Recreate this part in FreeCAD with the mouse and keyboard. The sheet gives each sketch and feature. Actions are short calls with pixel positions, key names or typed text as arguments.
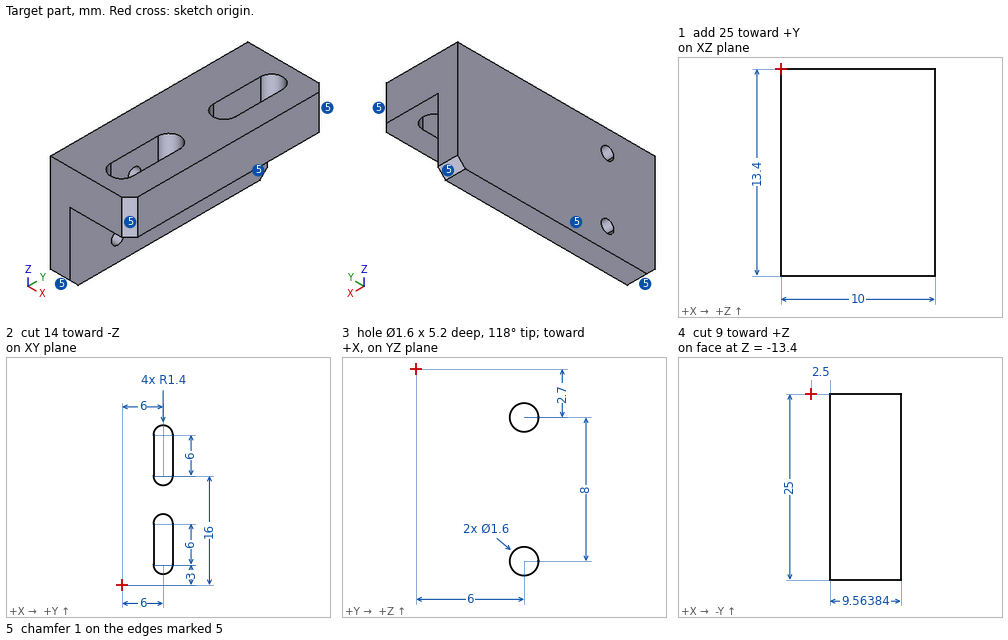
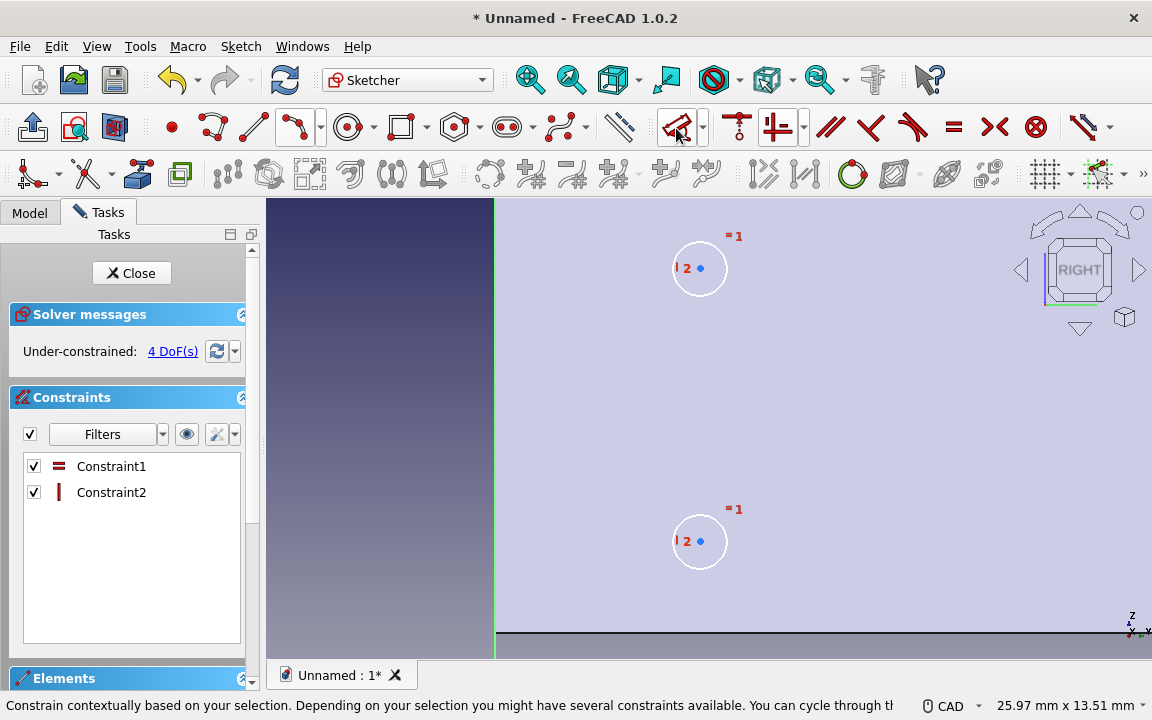
click(719, 523)
click(742, 500)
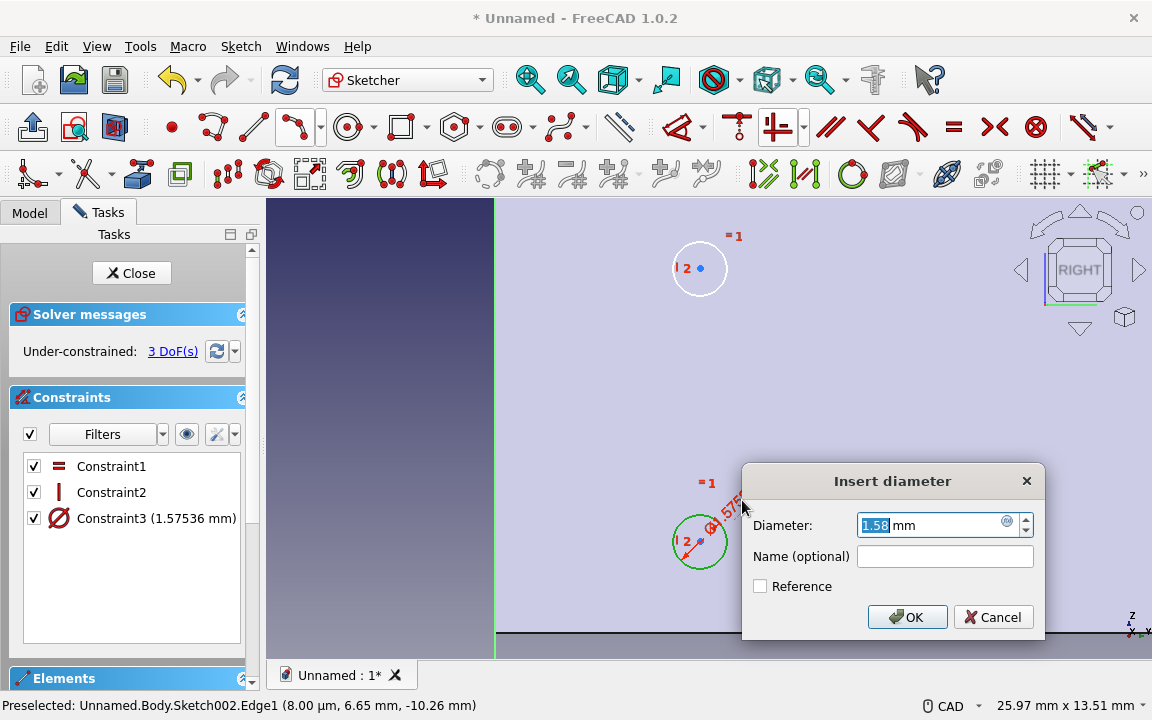
text(1.6)
key(Return)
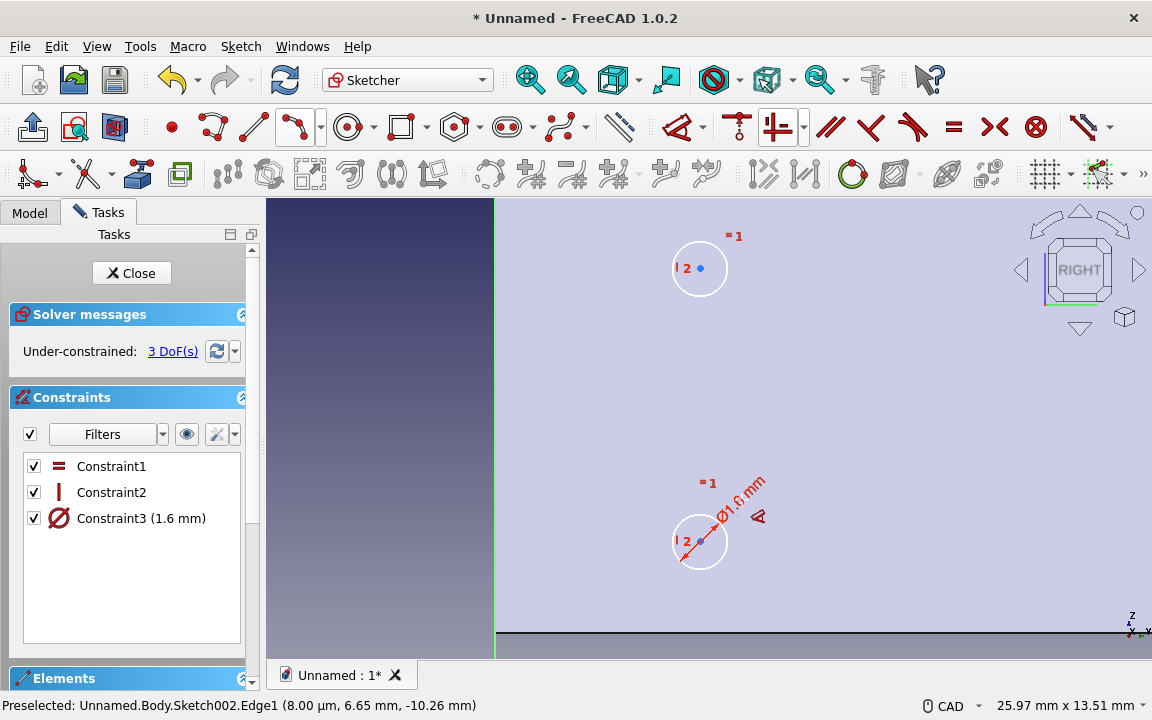
click(700, 542)
click(598, 576)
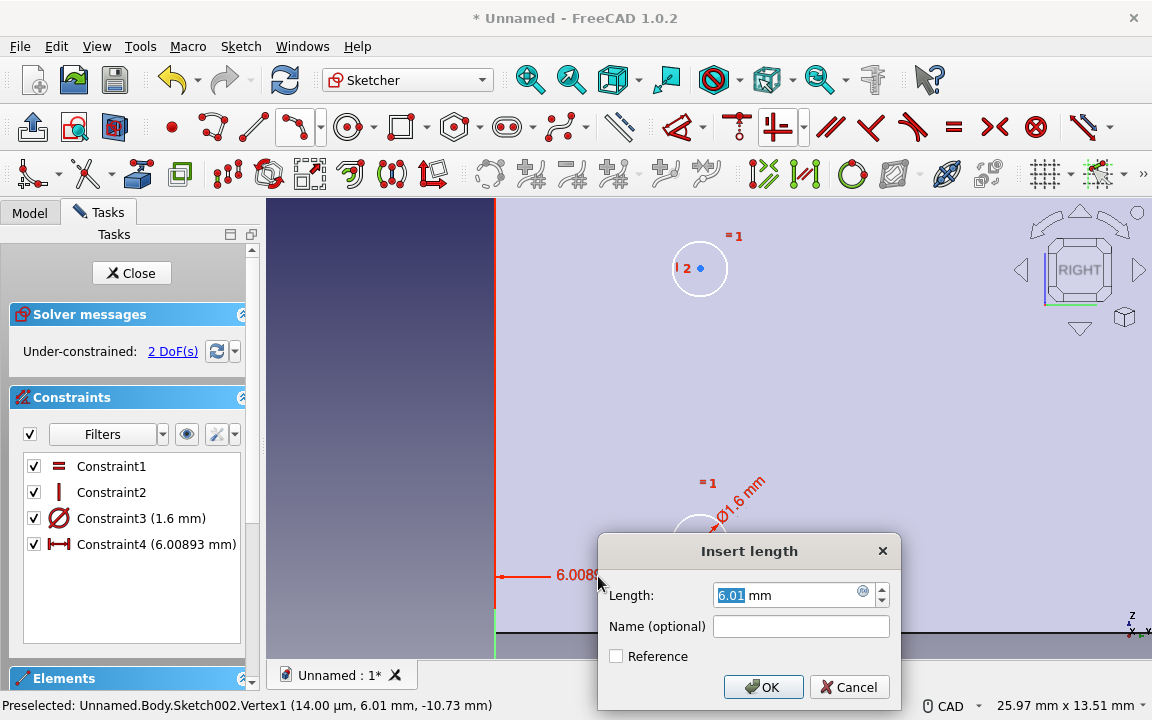
text(6)
key(Return)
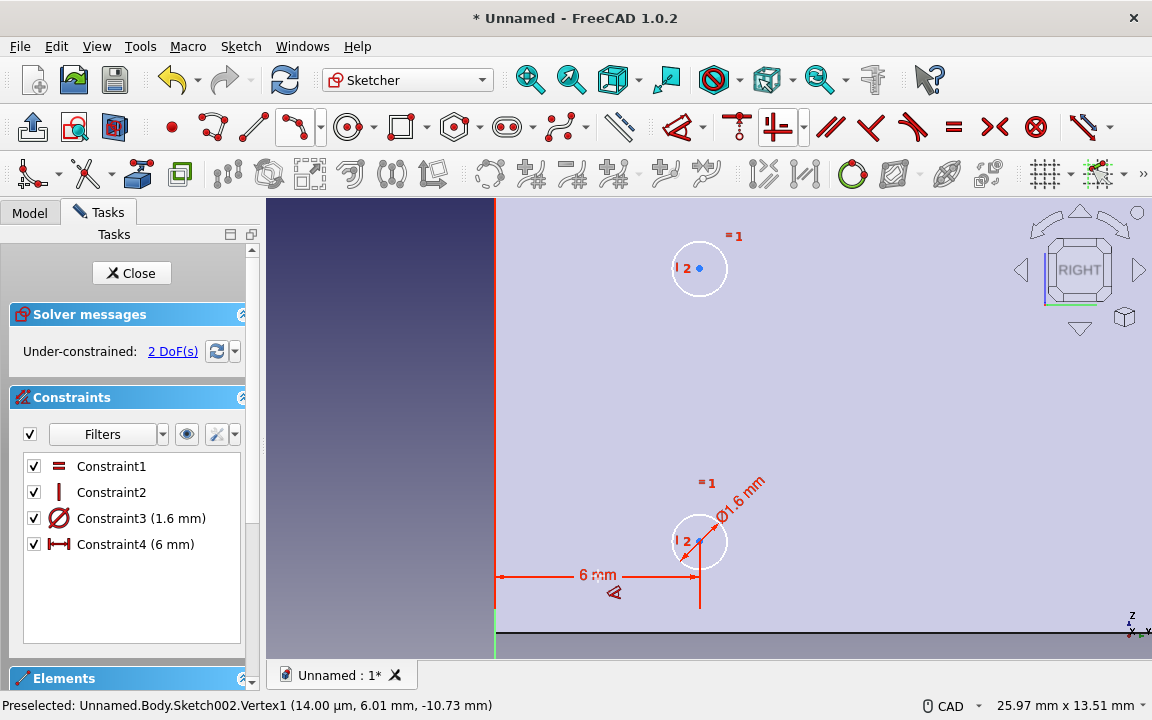
click(700, 542)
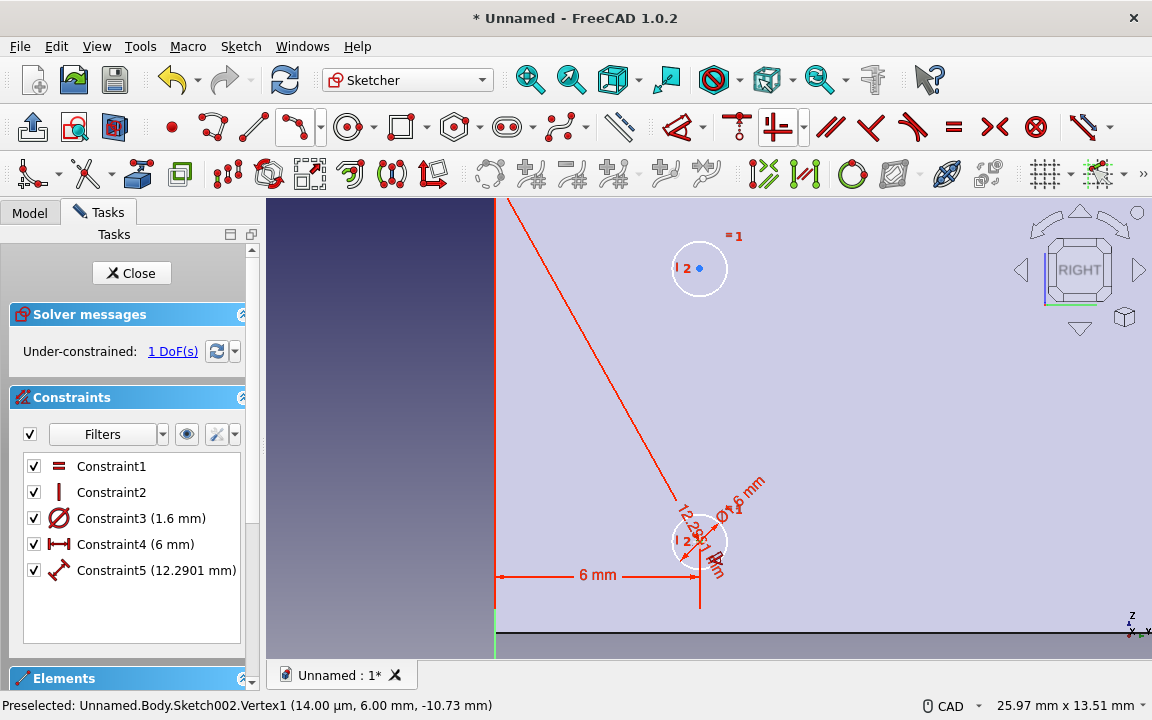
click(700, 269)
click(734, 406)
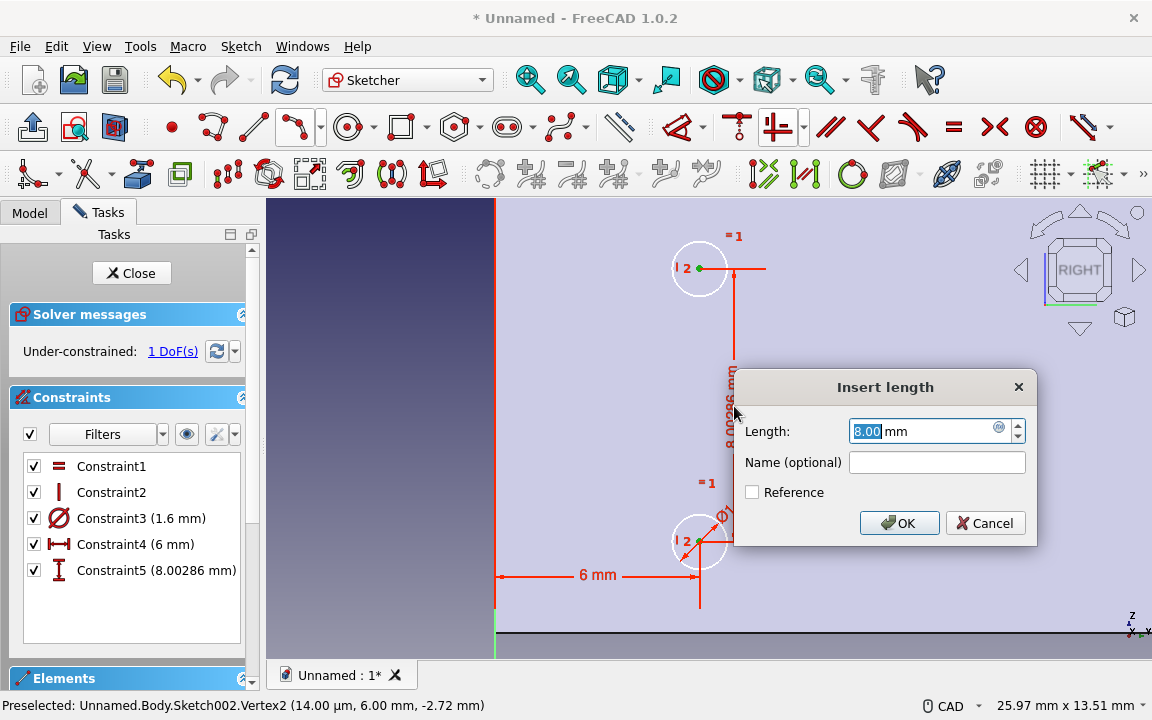
text(8)
key(Return)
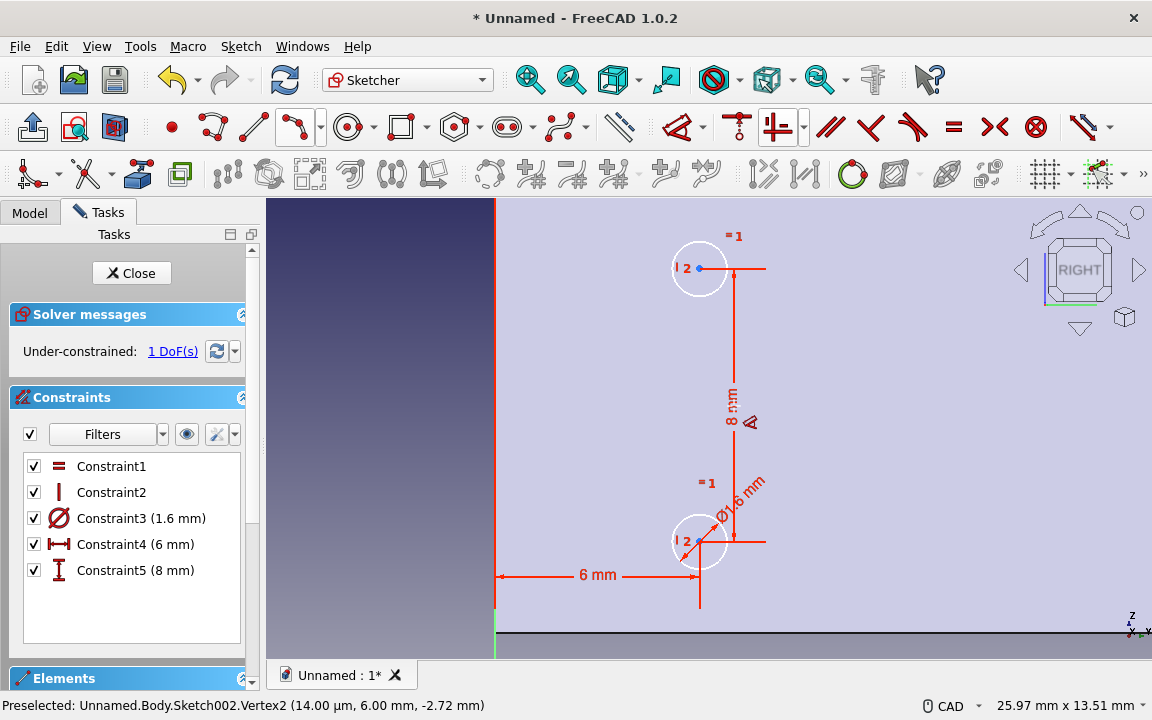
click(700, 269)
click(461, 247)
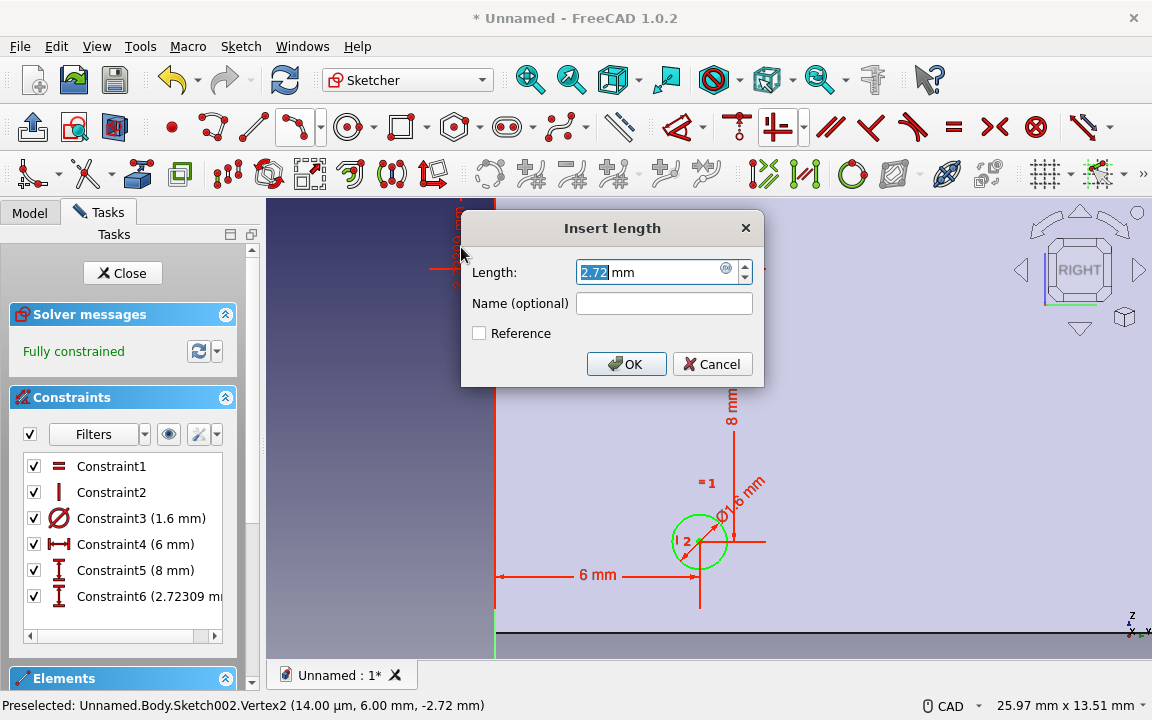
text(2.7)
key(Return)
key(Escape)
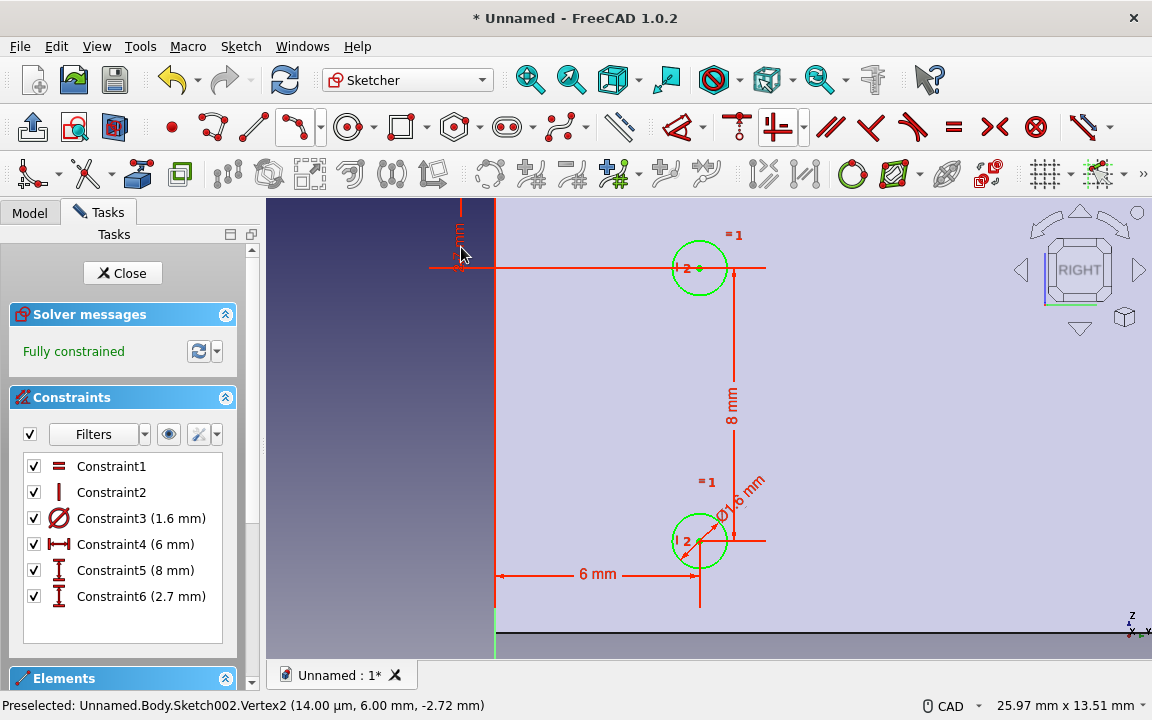
click(123, 273)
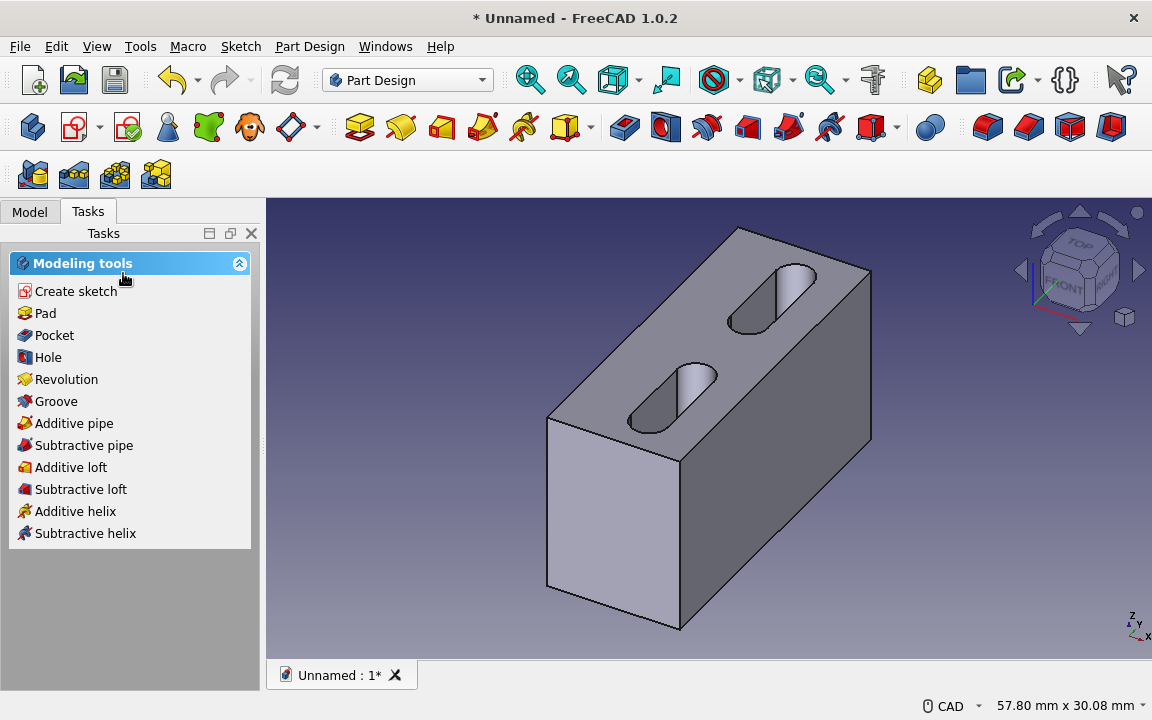
click(666, 128)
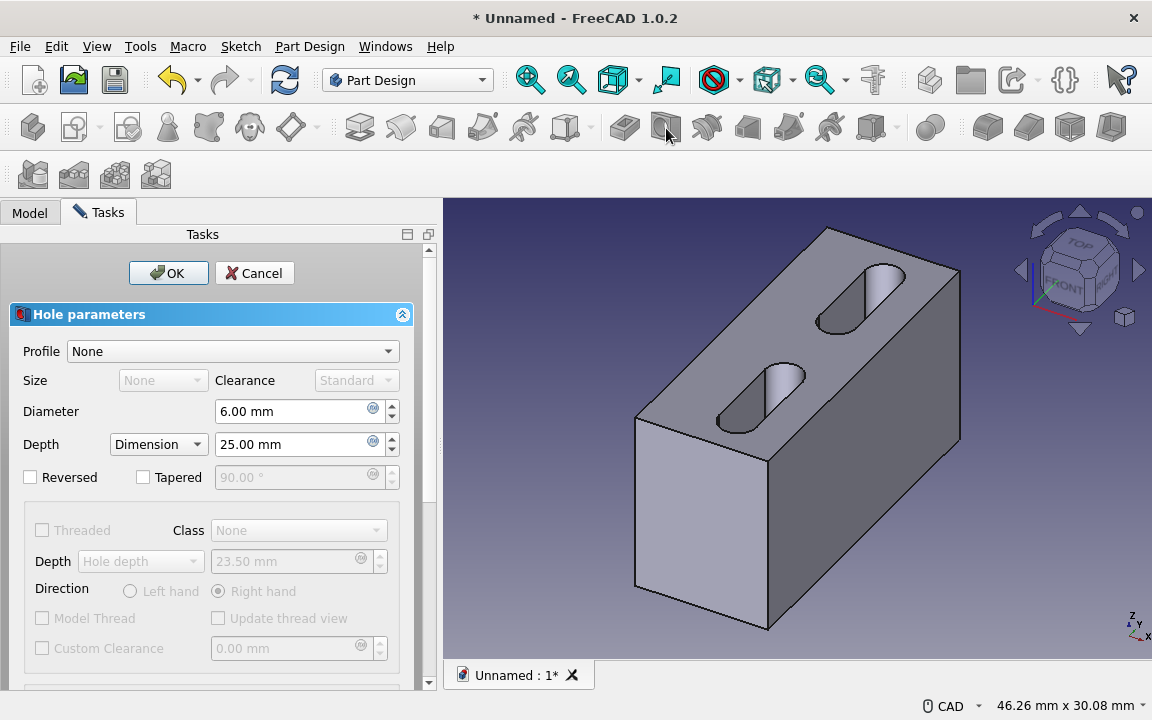
triple_click(300, 412)